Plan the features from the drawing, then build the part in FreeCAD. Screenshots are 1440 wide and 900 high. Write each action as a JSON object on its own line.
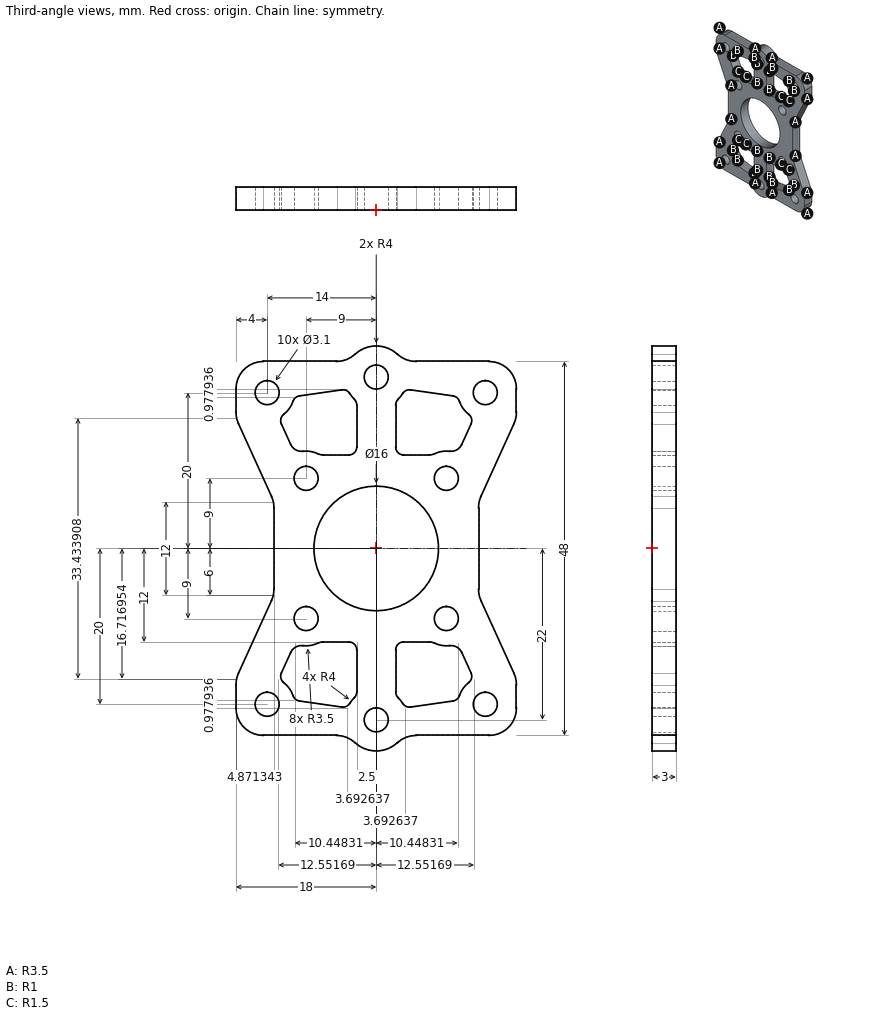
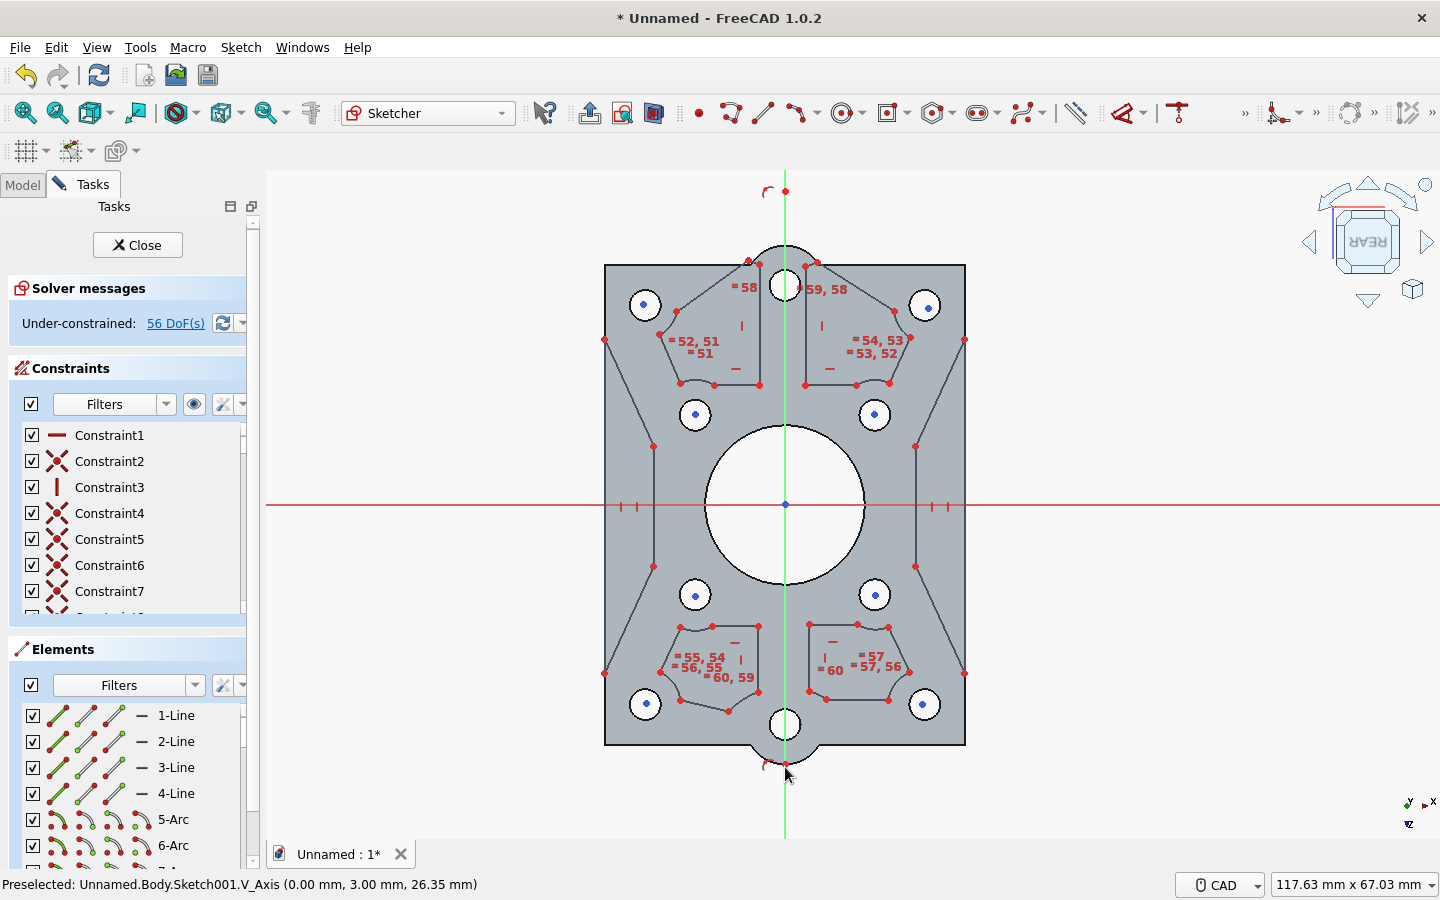
{"action": "left_click", "coordinate": [695, 414]}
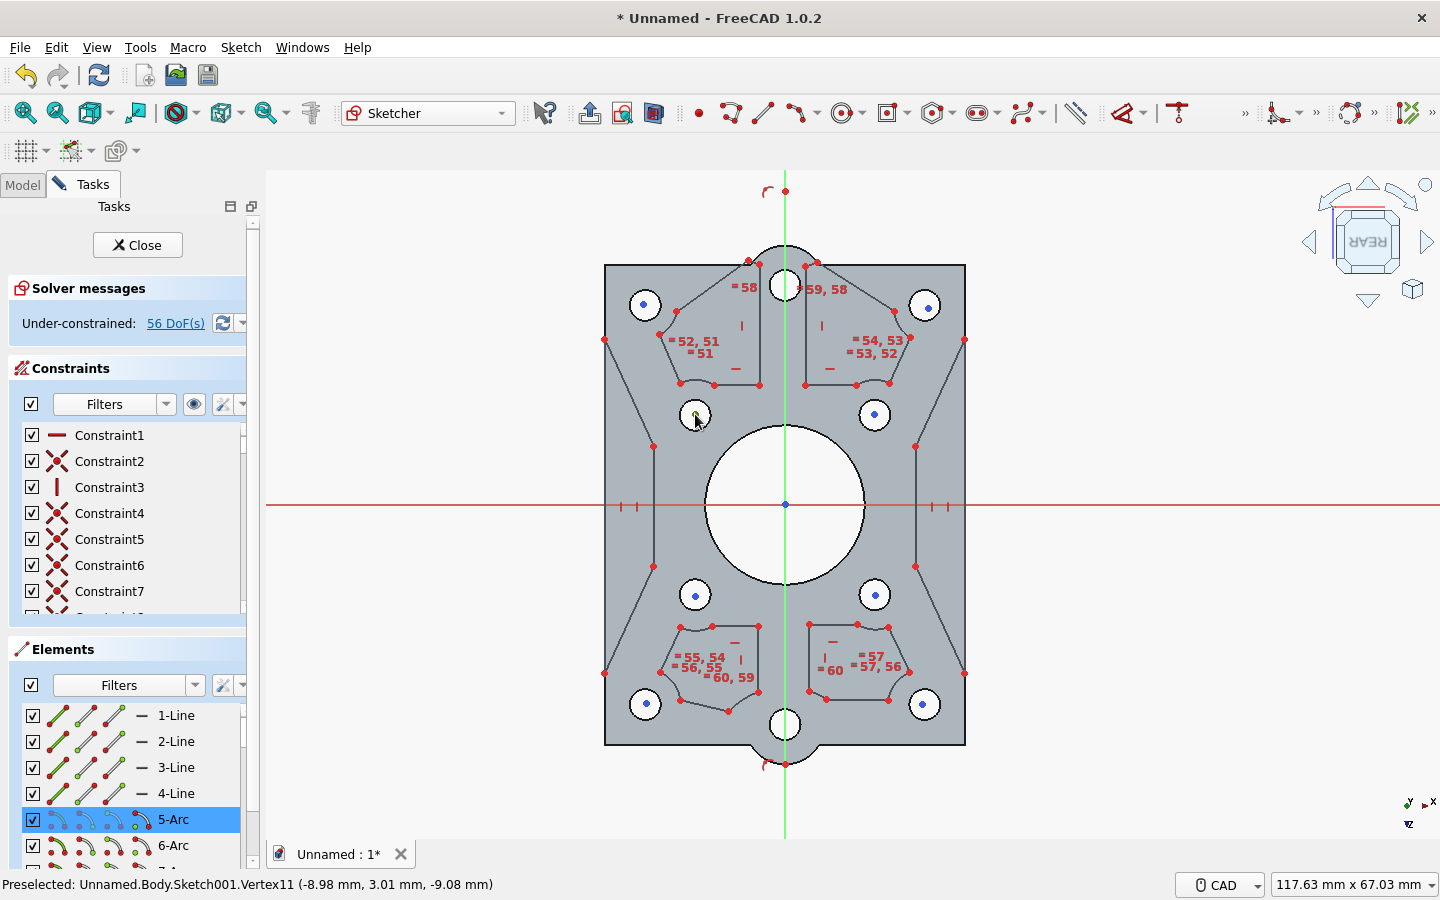
{"action": "left_click", "coordinate": [875, 414]}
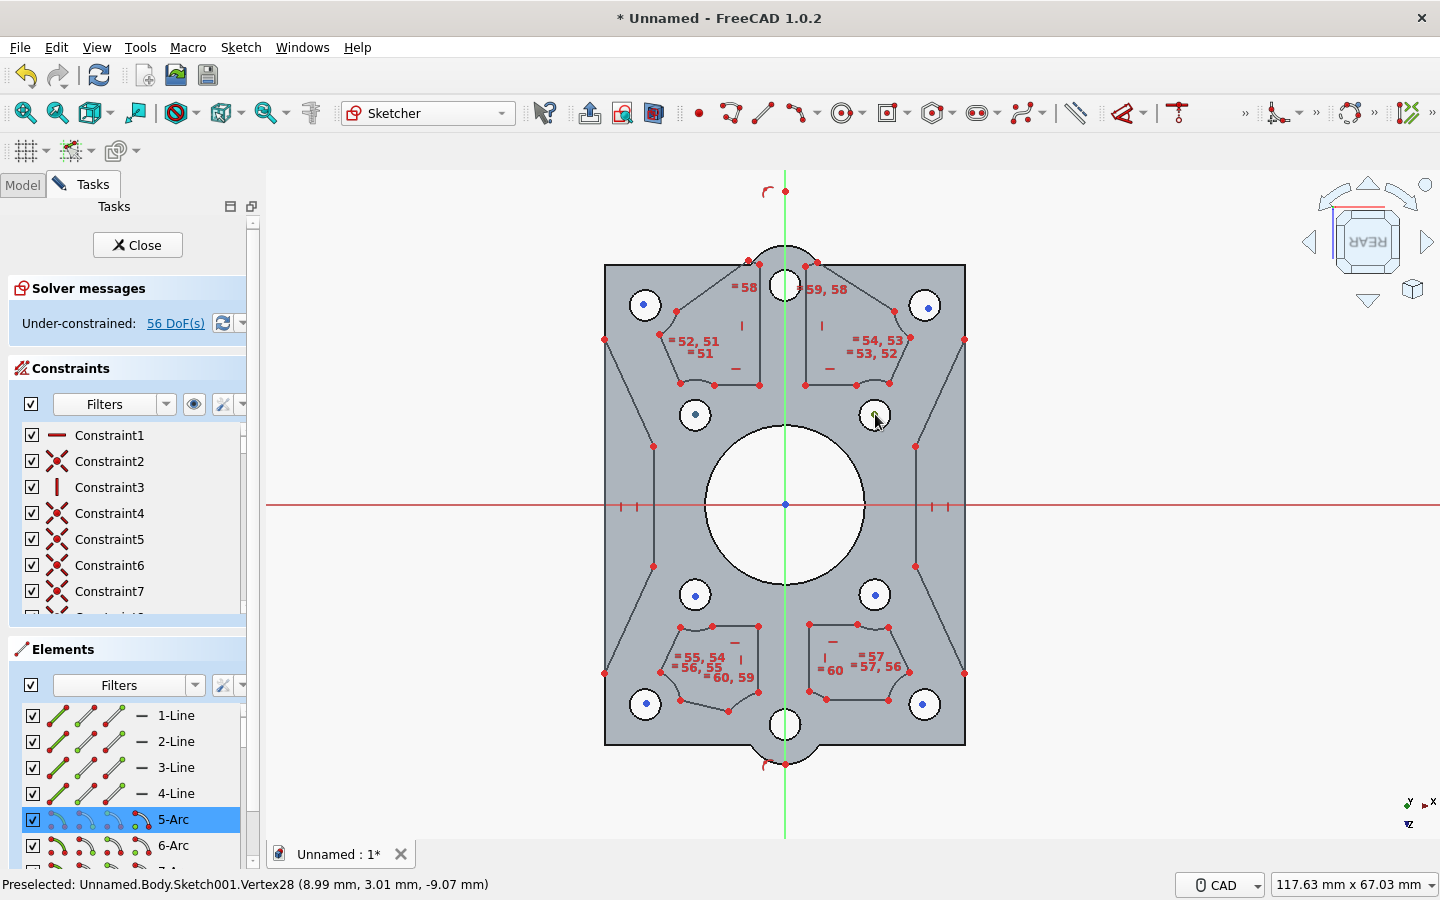
{"action": "left_click", "coordinate": [785, 723]}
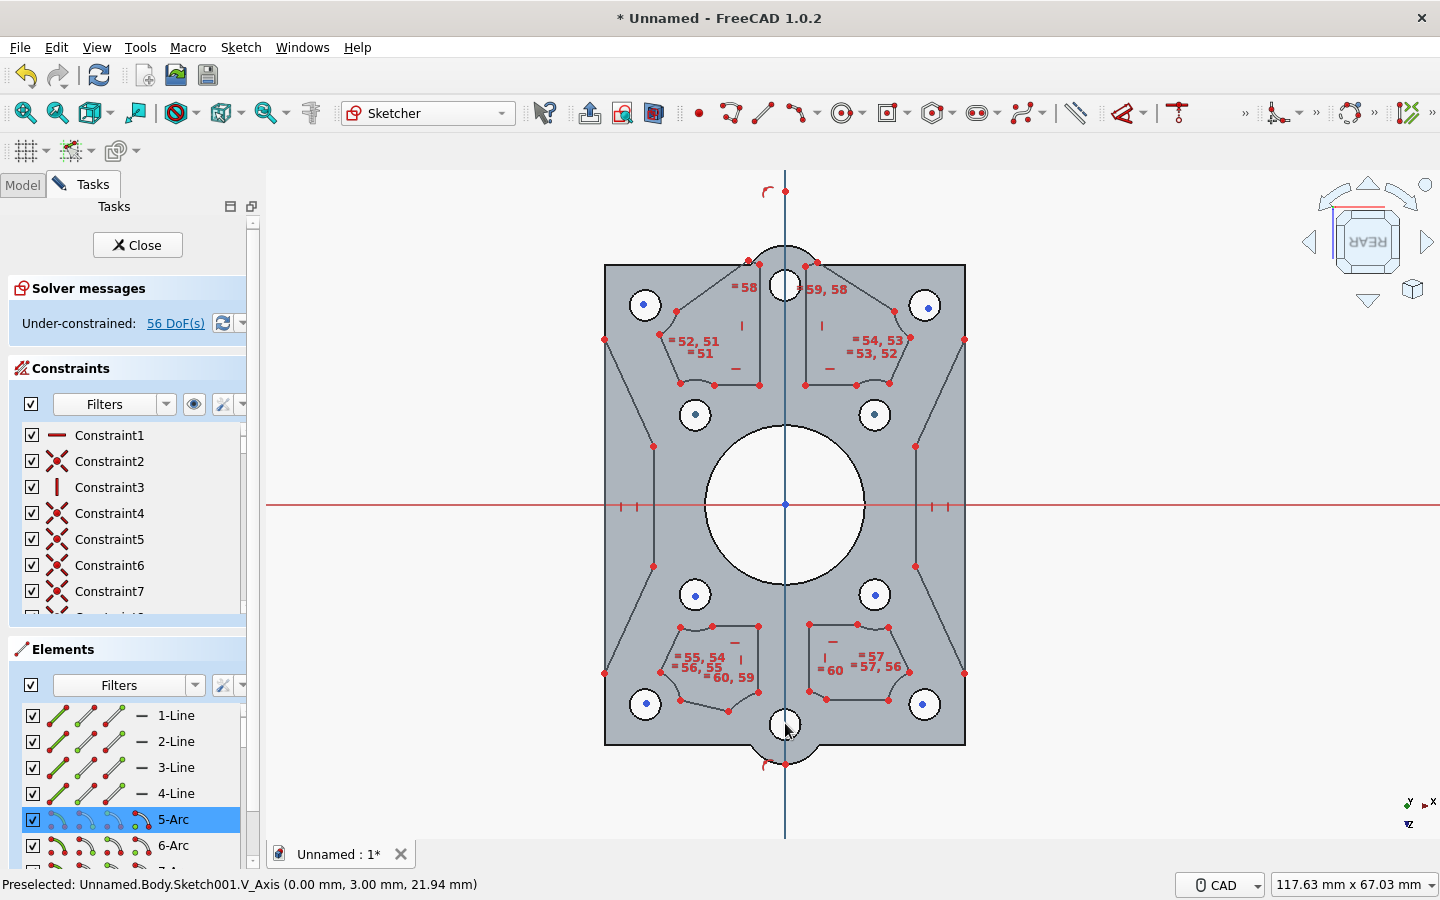
{"action": "key", "text": "s"}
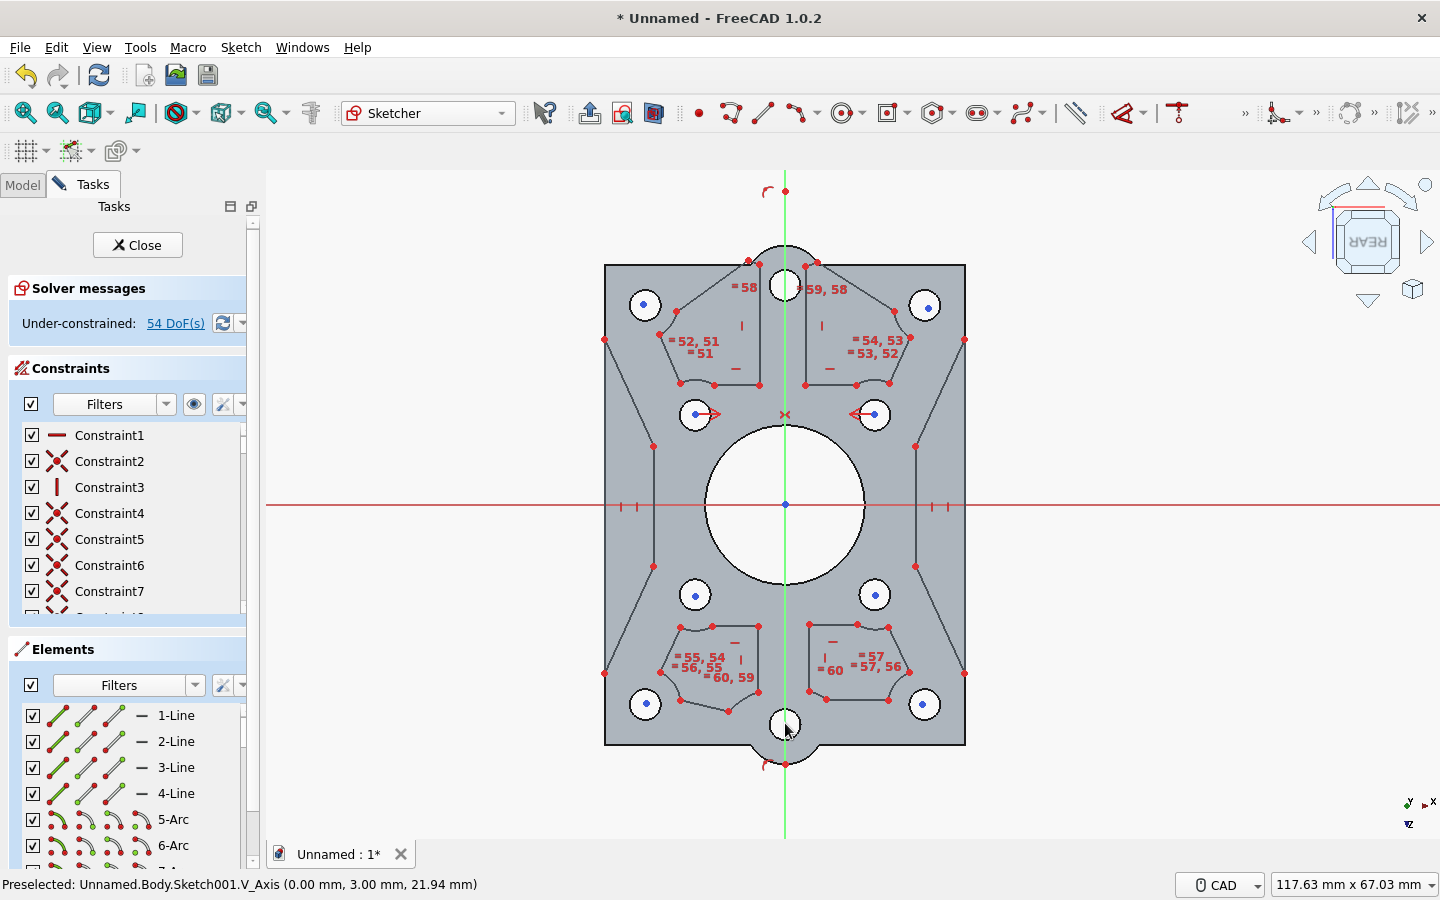
{"action": "left_click", "coordinate": [643, 305]}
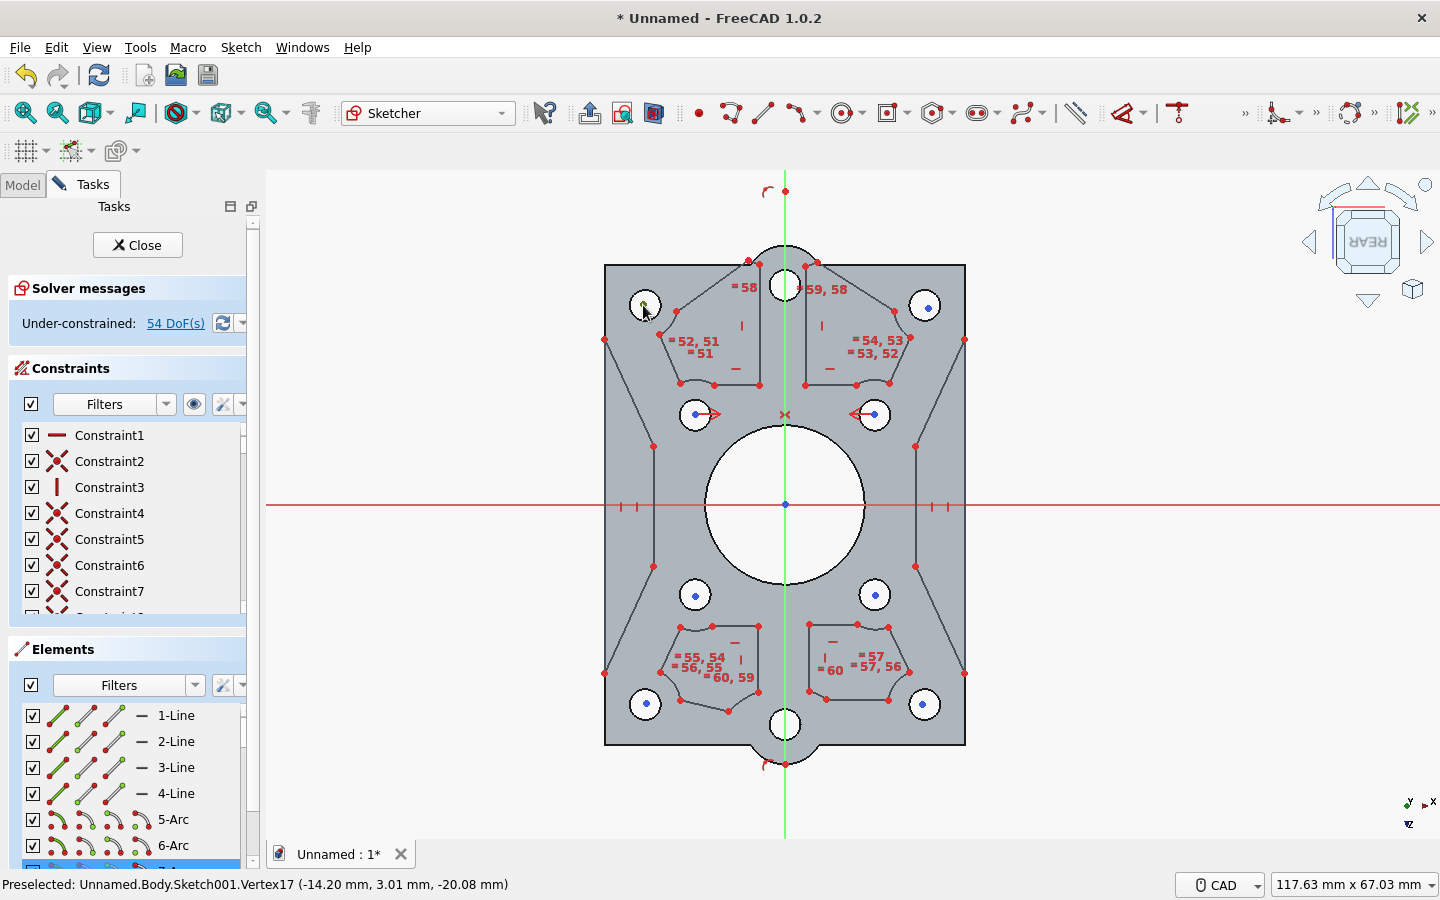
{"action": "left_click", "coordinate": [929, 308]}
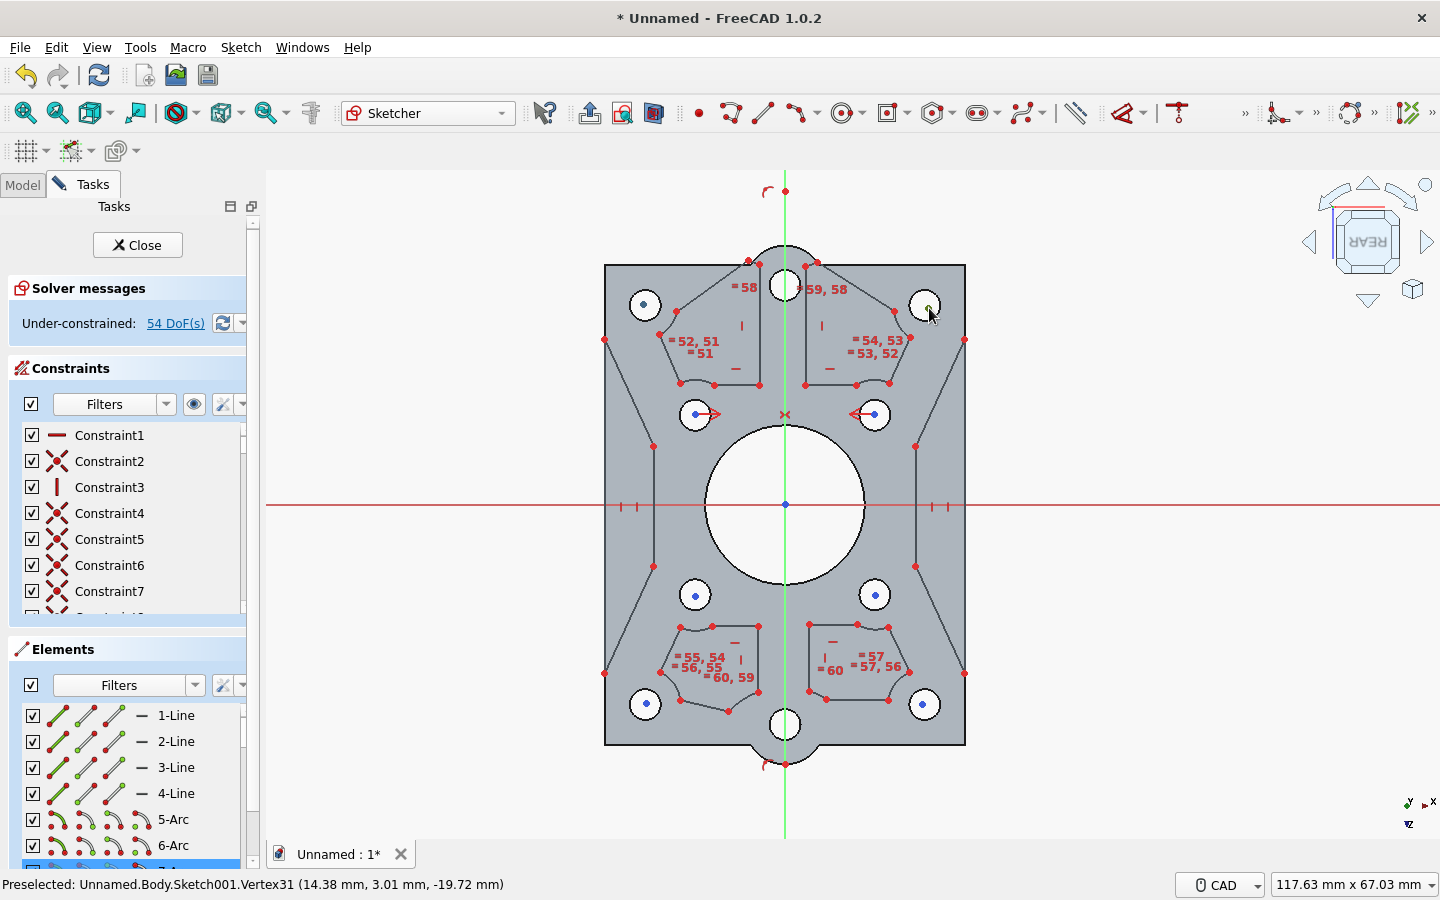
{"action": "left_click", "coordinate": [785, 723]}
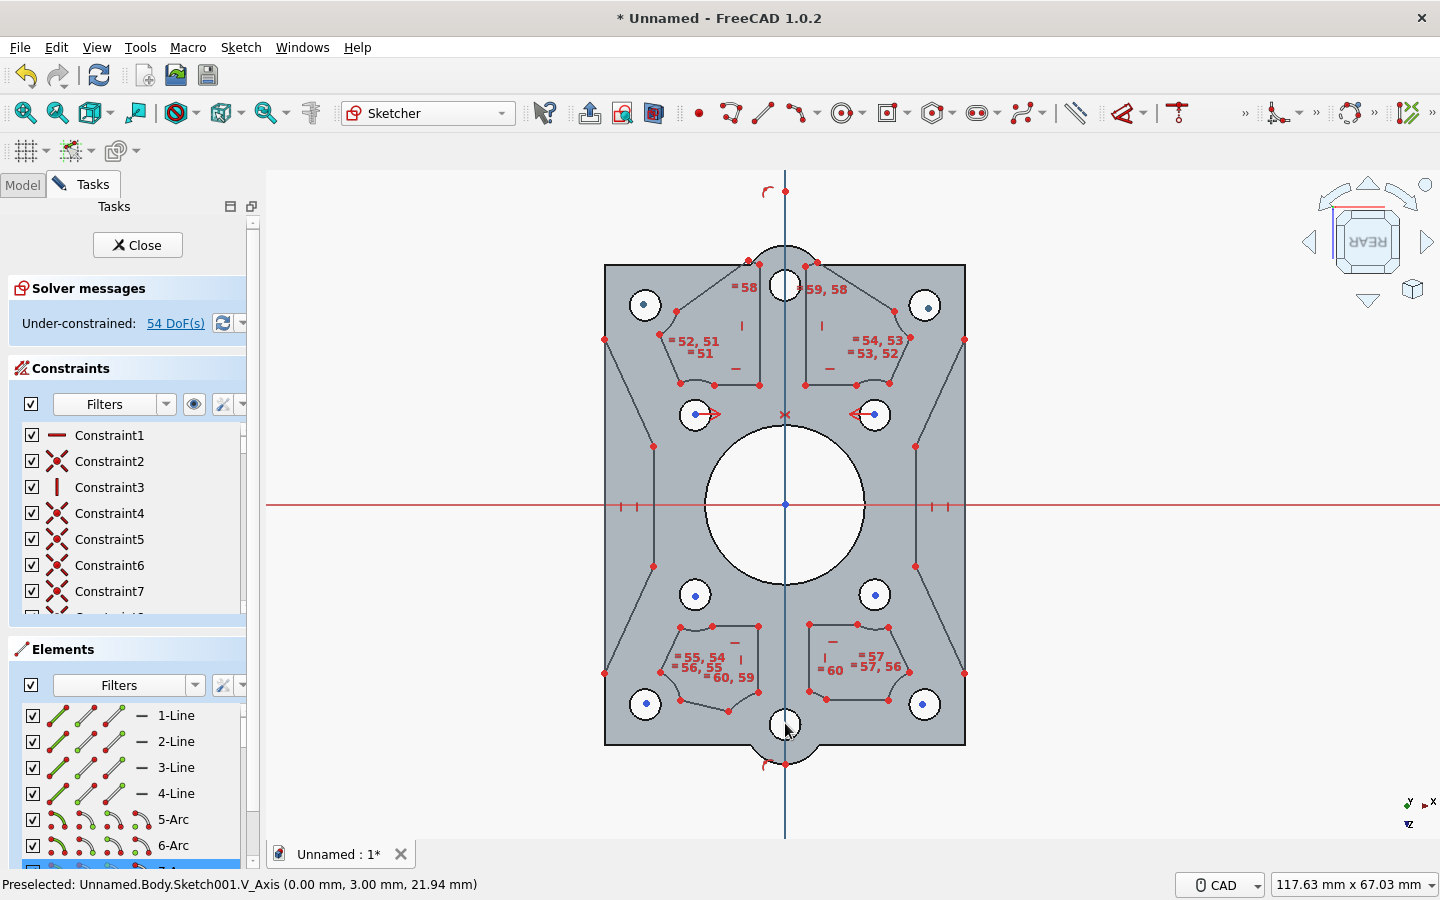
{"action": "key", "text": "s"}